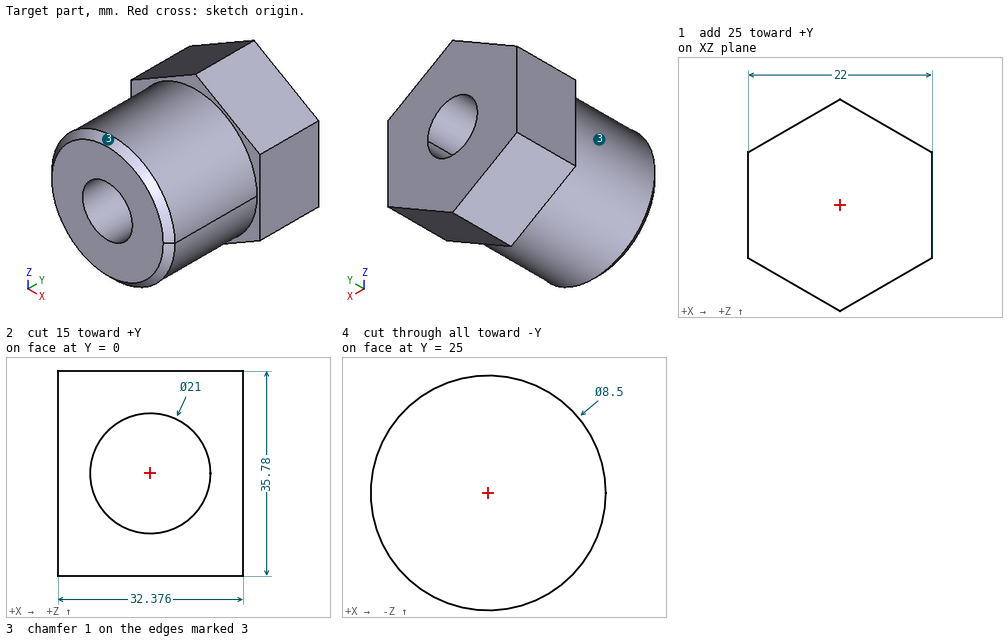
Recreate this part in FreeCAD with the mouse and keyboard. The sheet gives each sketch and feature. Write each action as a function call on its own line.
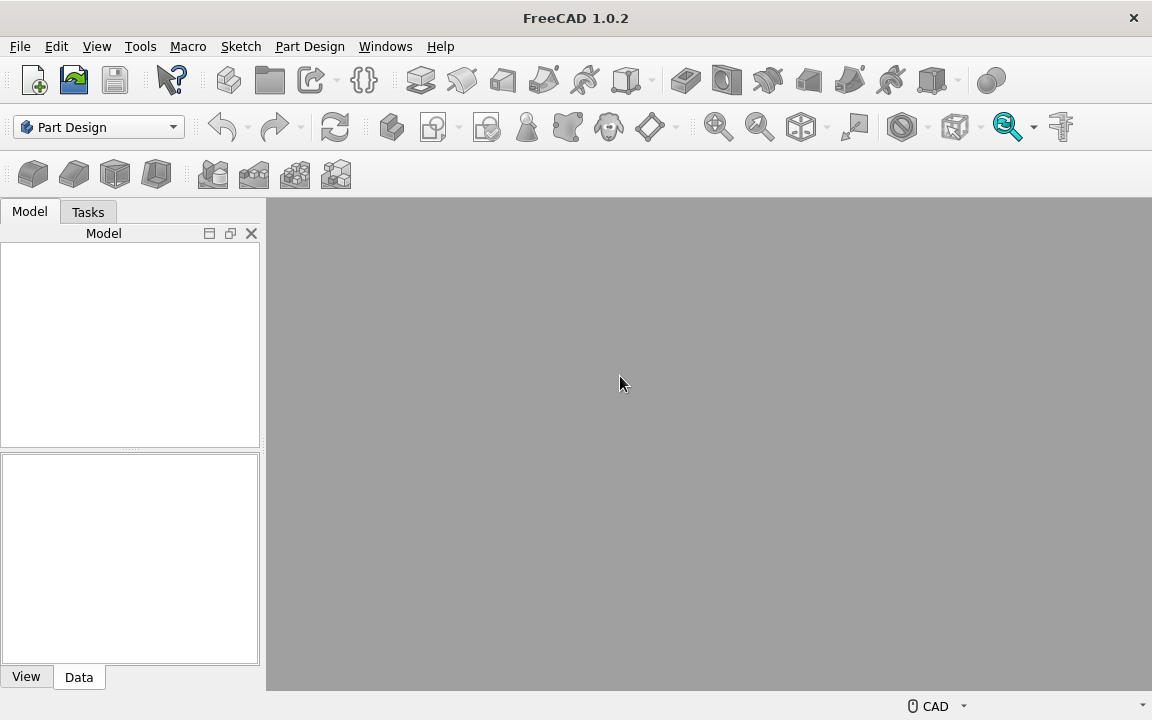
key(ctrl+n)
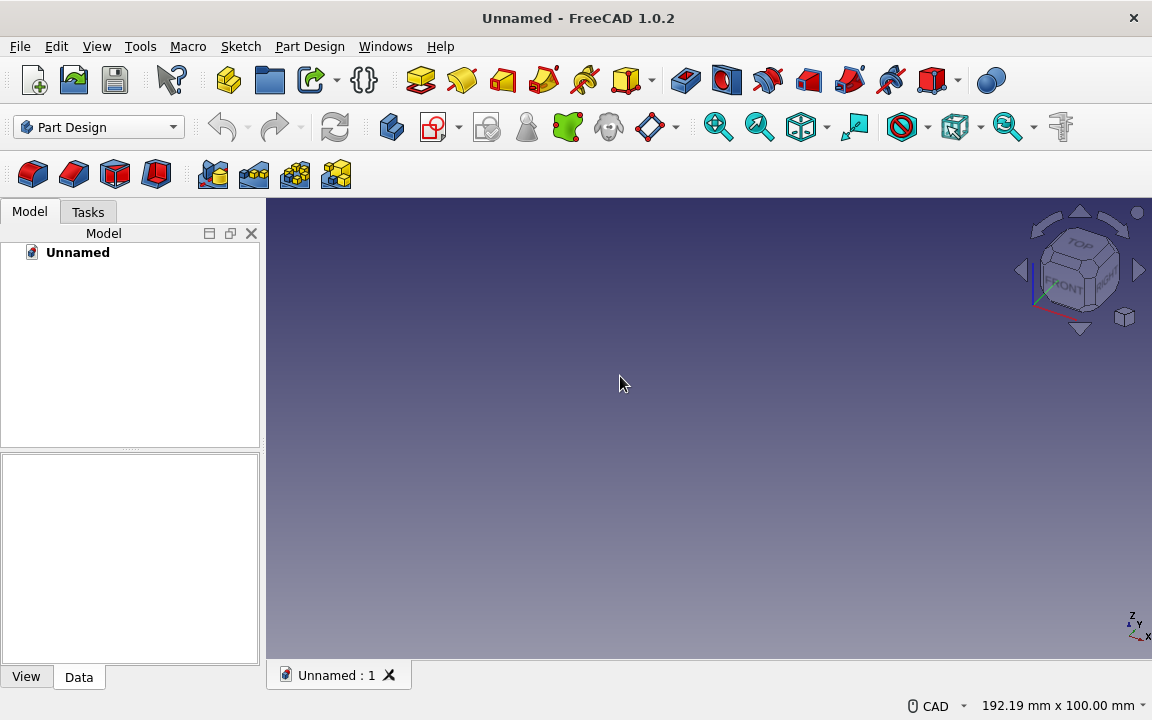
click(432, 128)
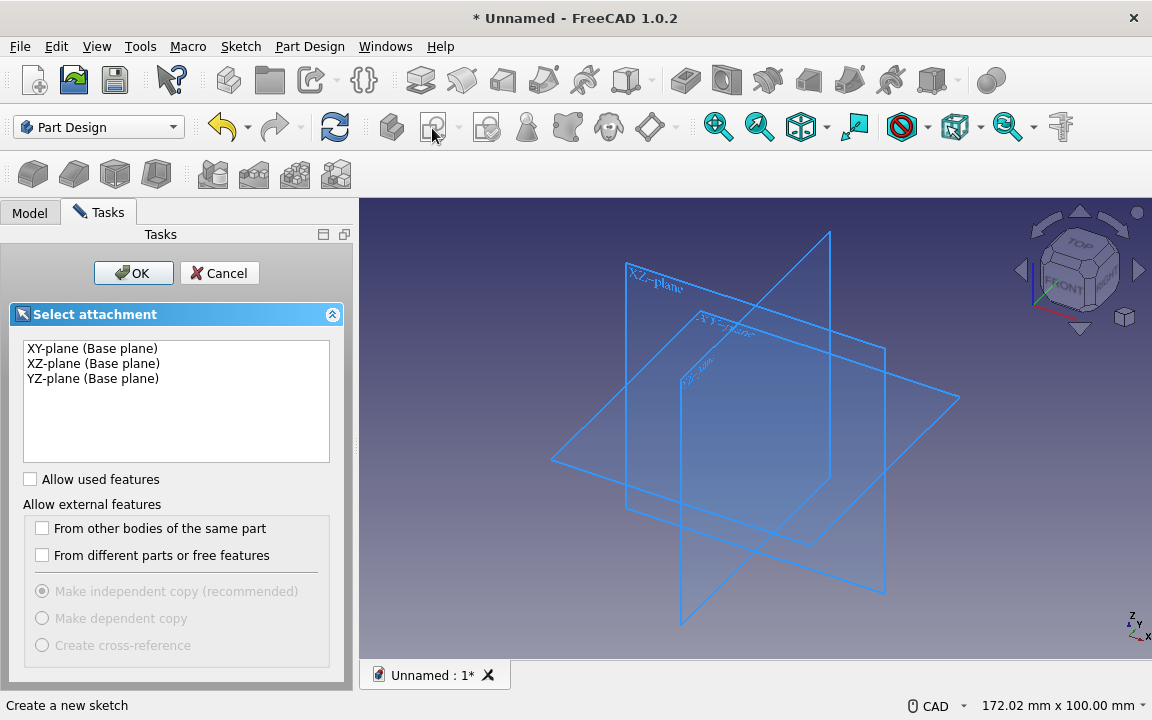
click(84, 364)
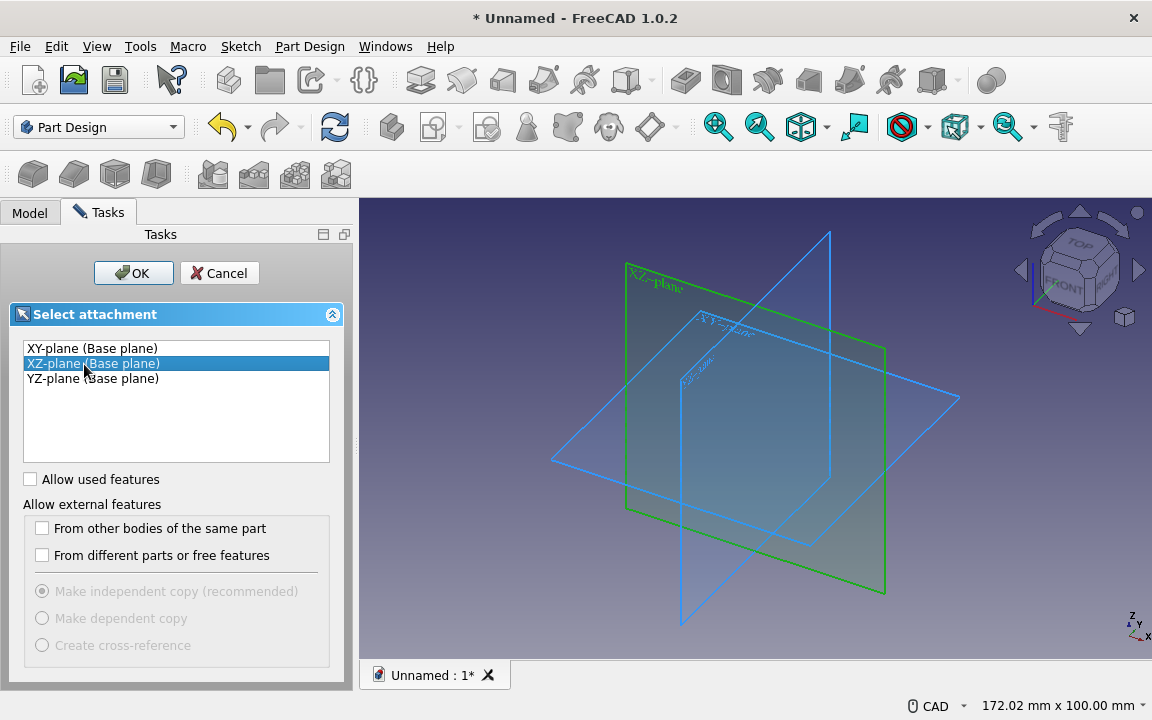
click(134, 273)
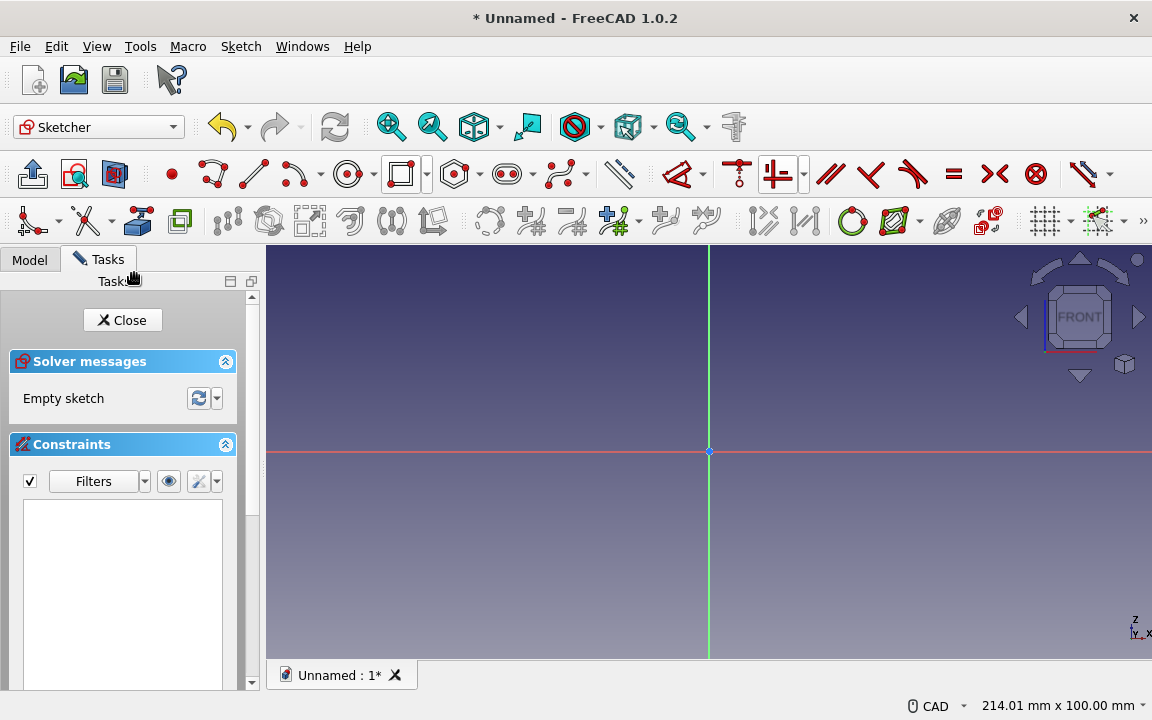
scroll(765, 452, up, 4)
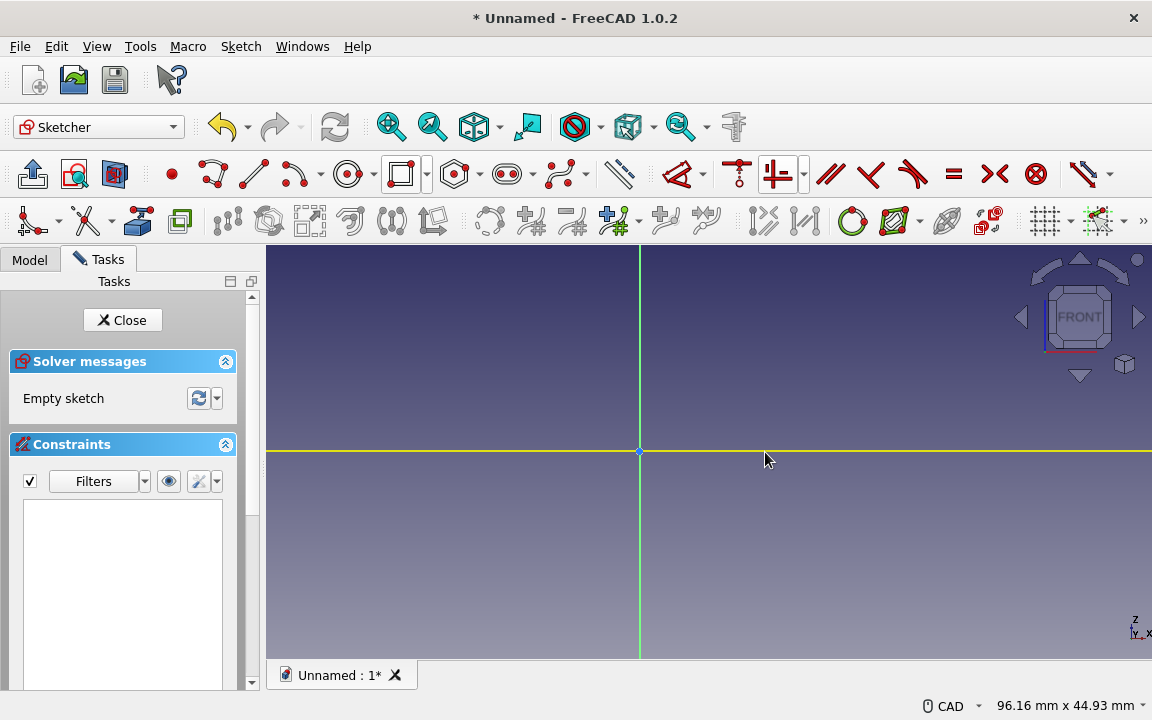
key(g)
key(p)
key(6)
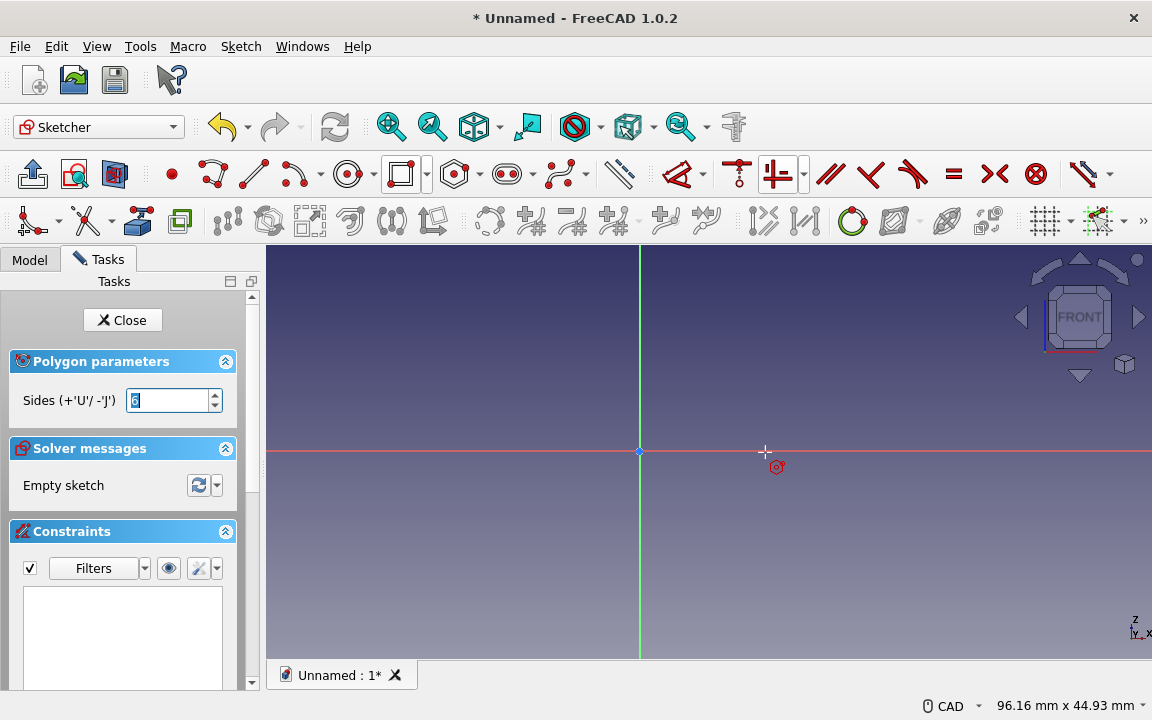
click(640, 451)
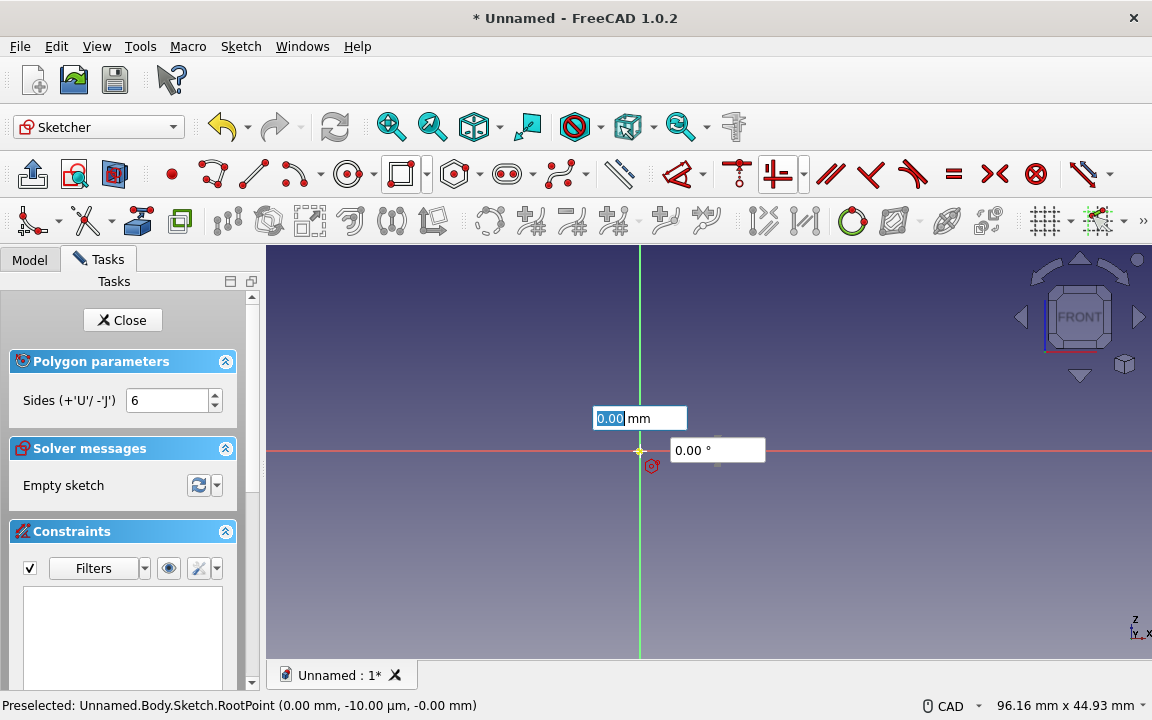
click(640, 568)
right_click(640, 568)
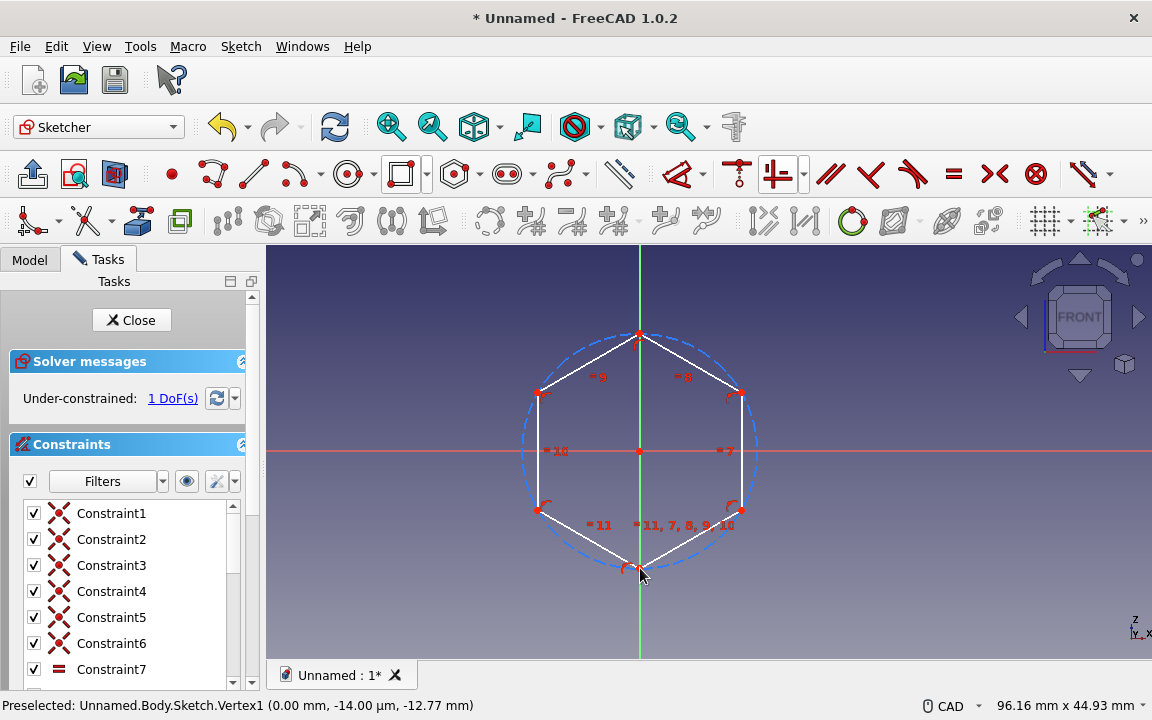
key(d)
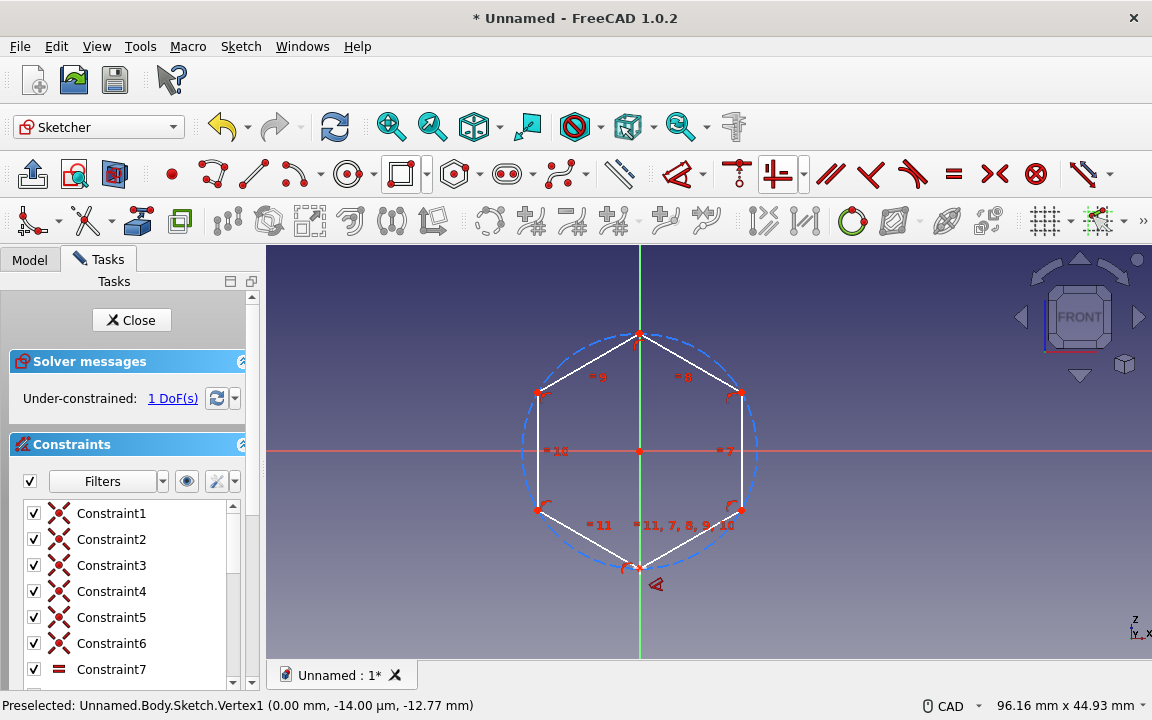
click(538, 393)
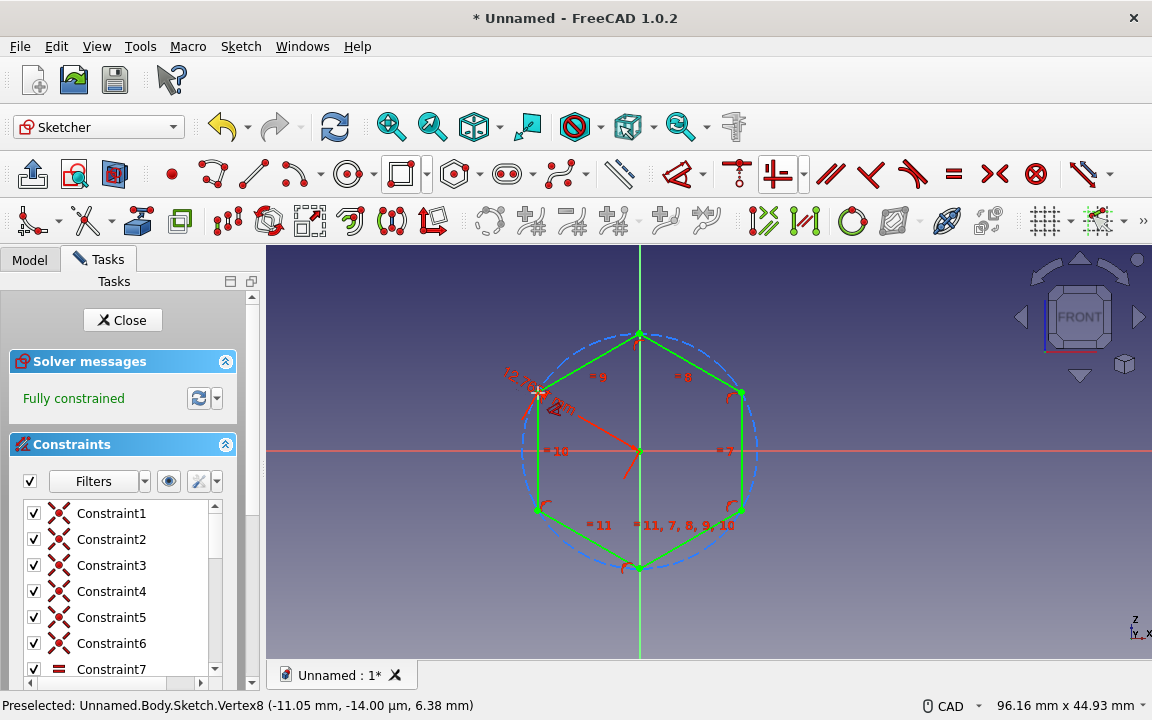
click(742, 510)
click(568, 335)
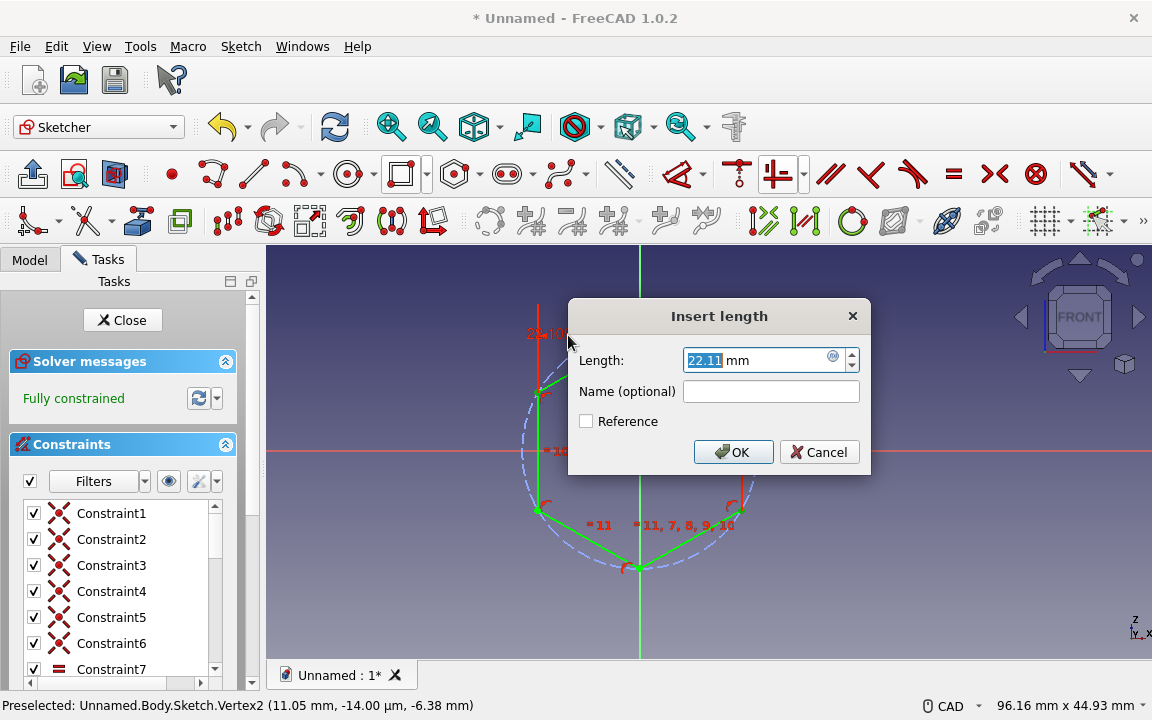
text(22)
key(Return)
key(Escape)